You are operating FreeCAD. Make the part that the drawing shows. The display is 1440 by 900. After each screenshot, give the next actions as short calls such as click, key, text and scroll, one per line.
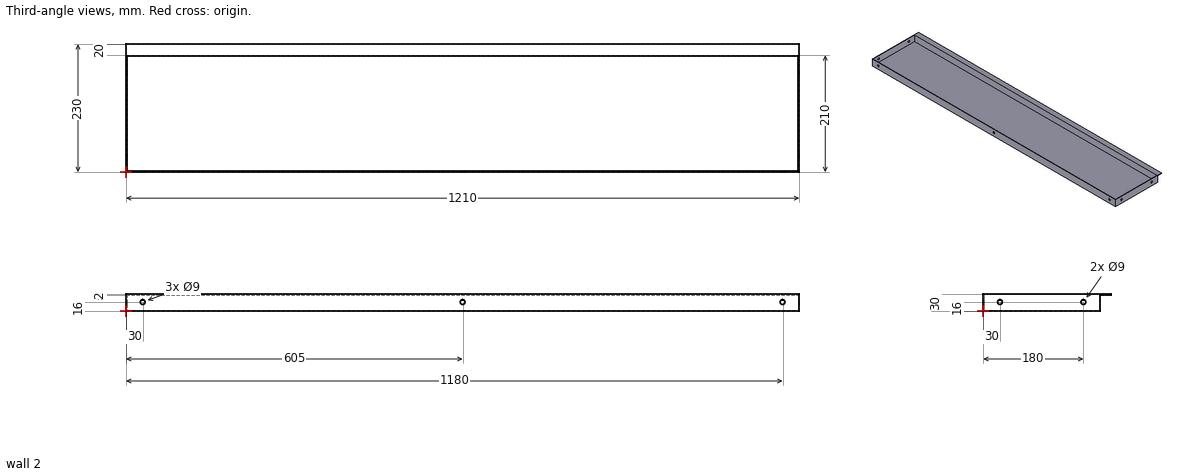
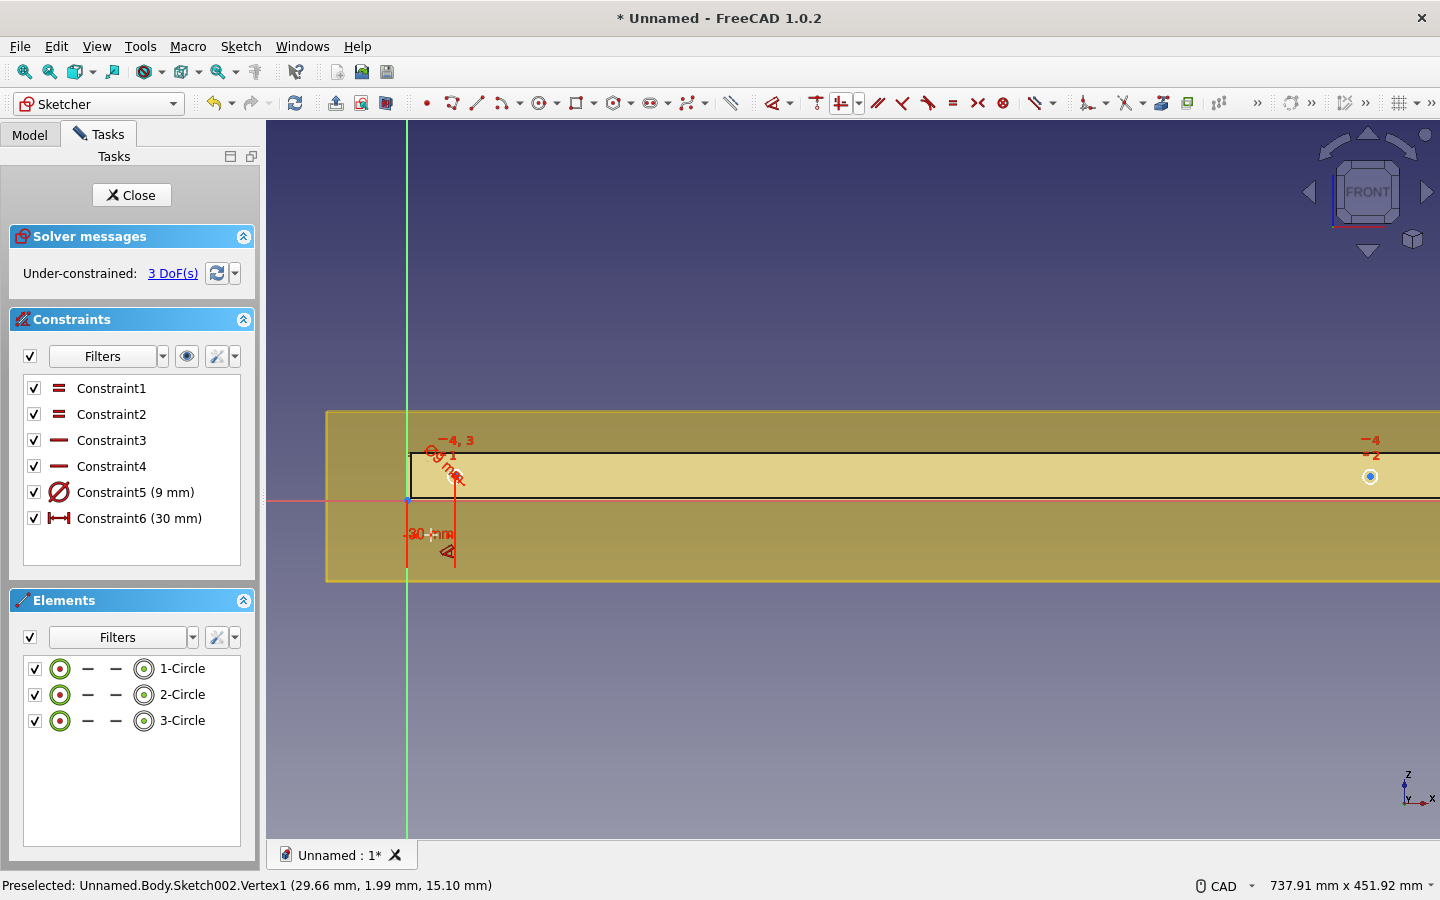
scroll(455, 477, up, 3)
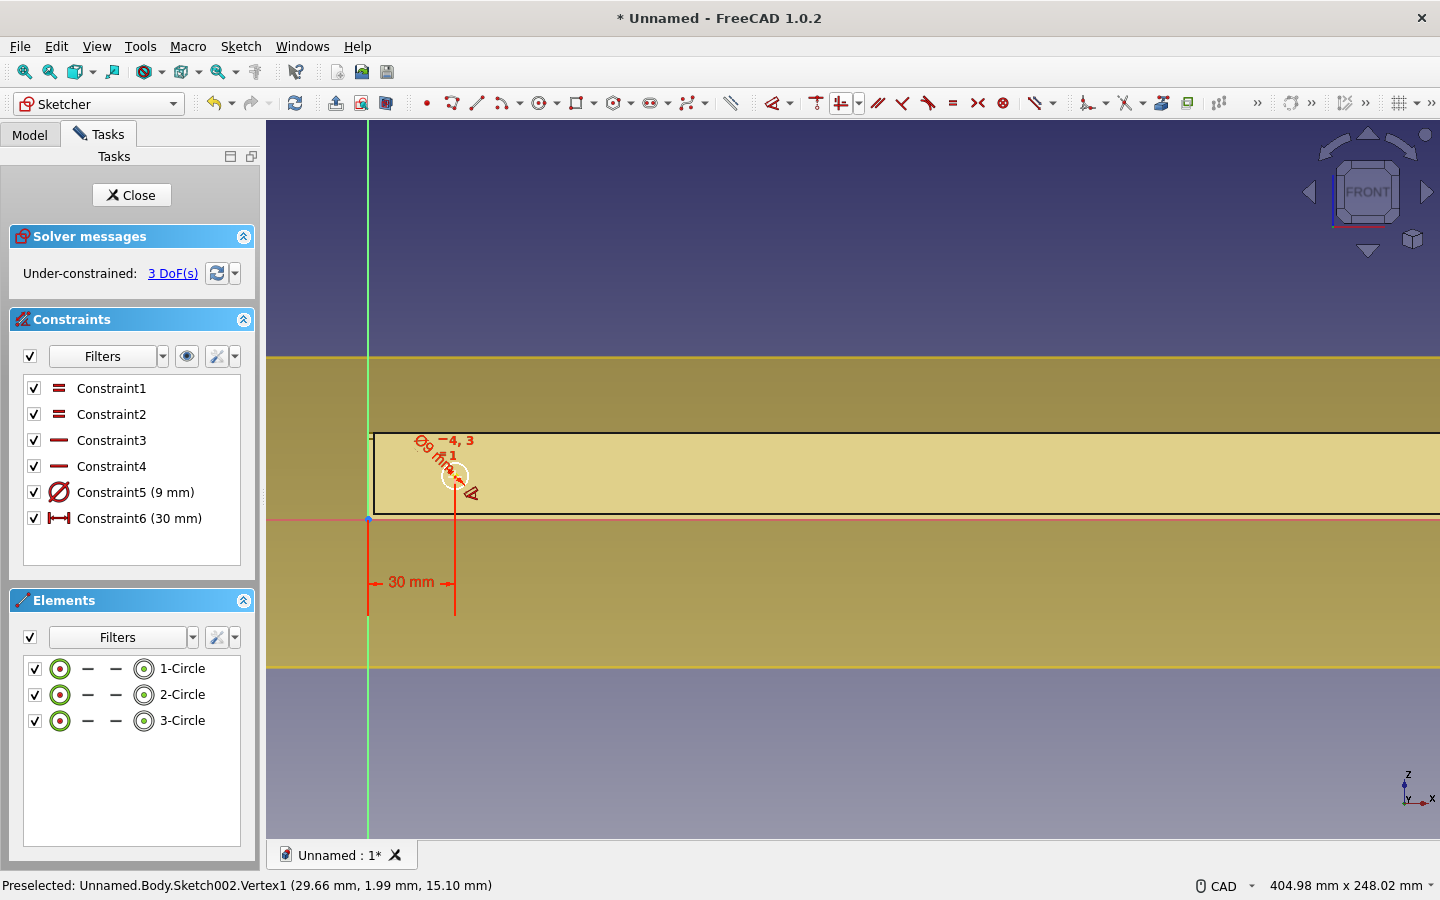
click(455, 476)
click(334, 498)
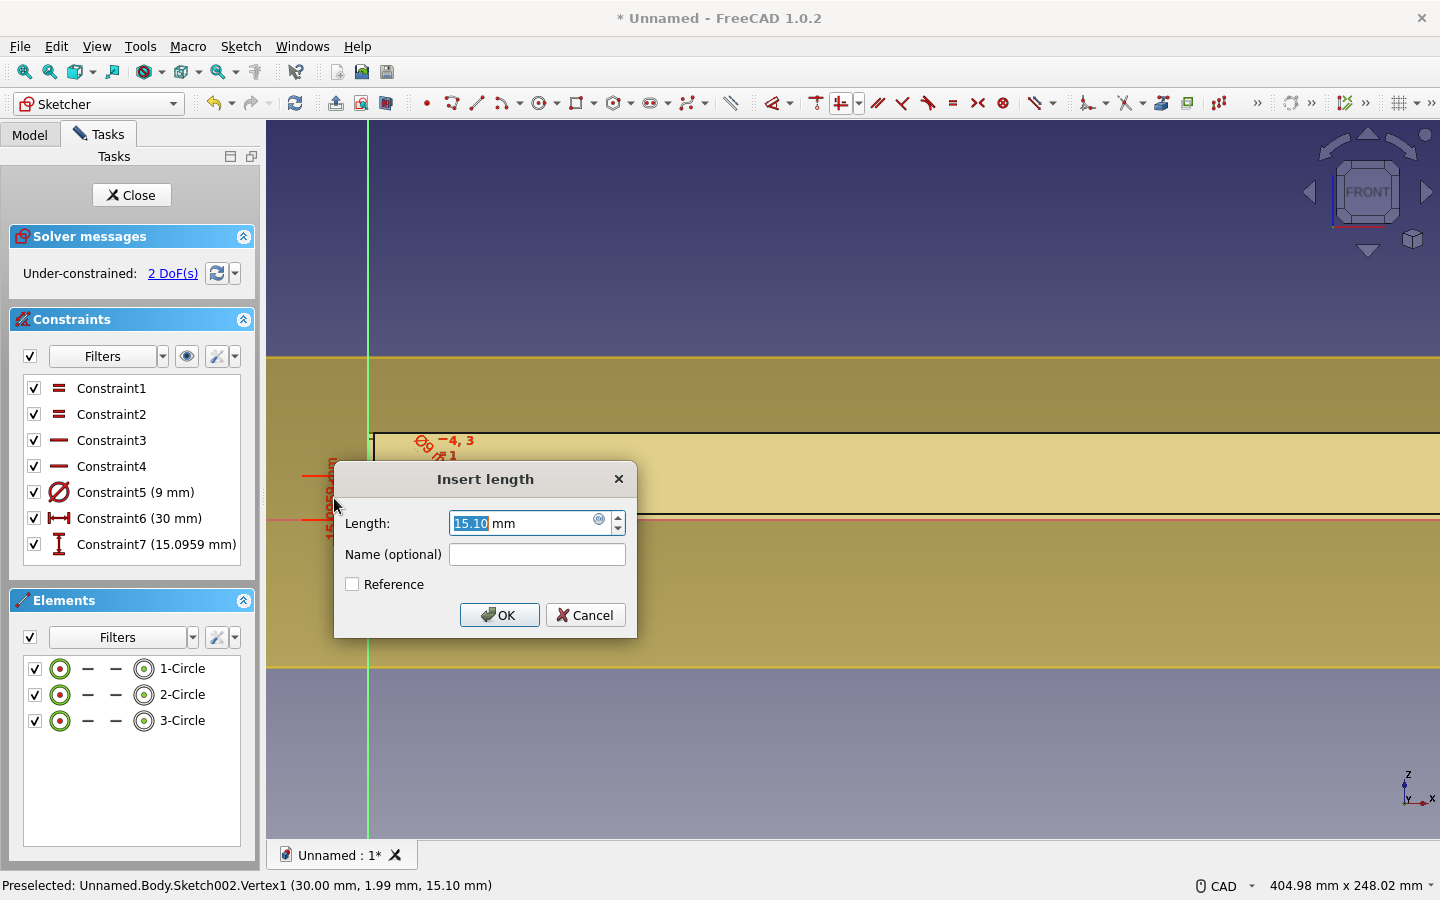
text(16)
key(Return)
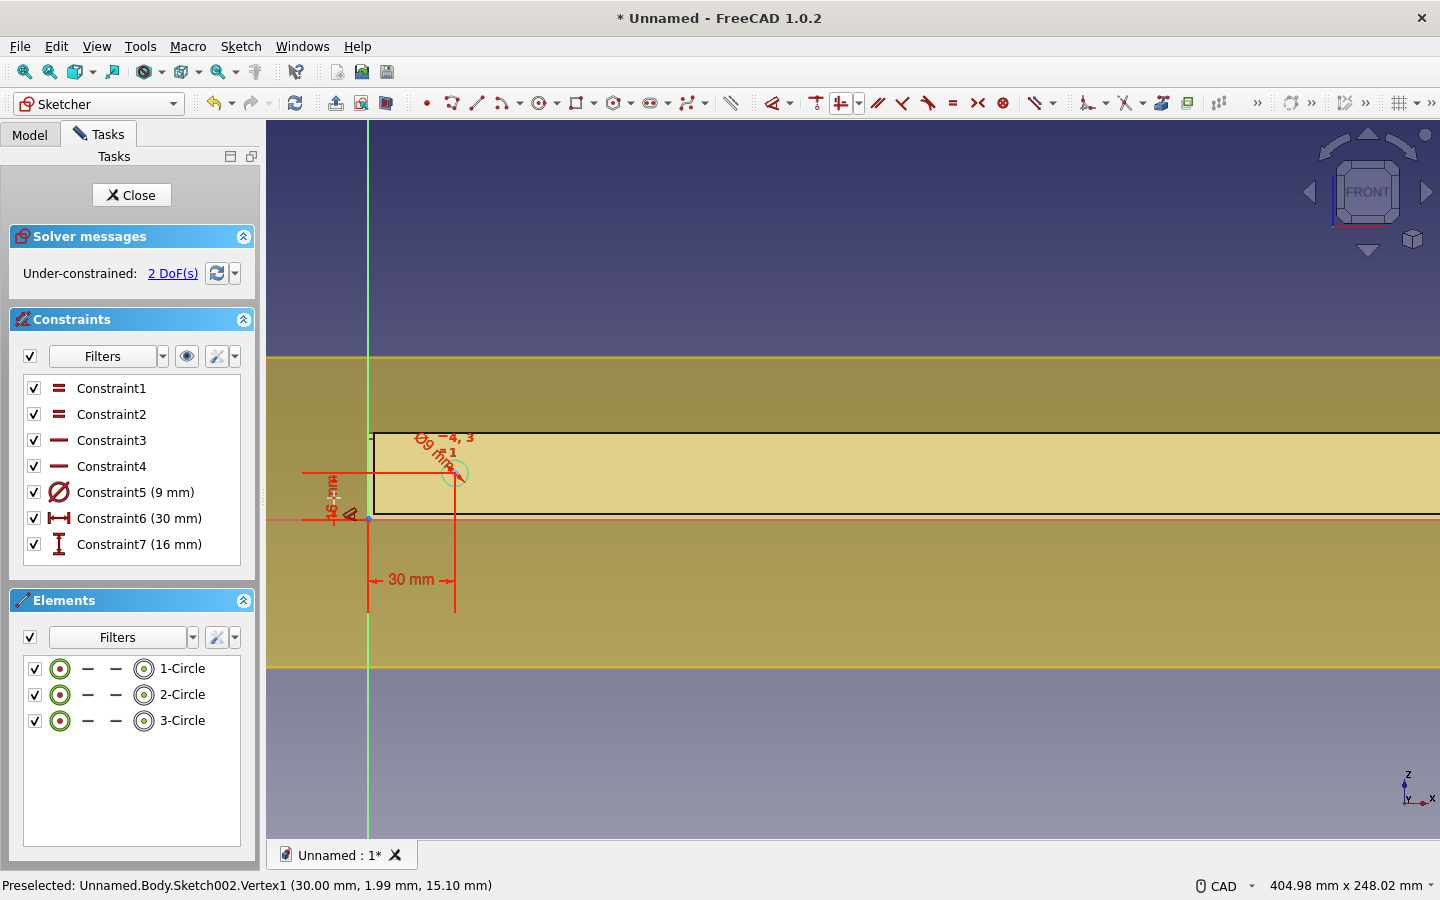
scroll(455, 477, down, 8)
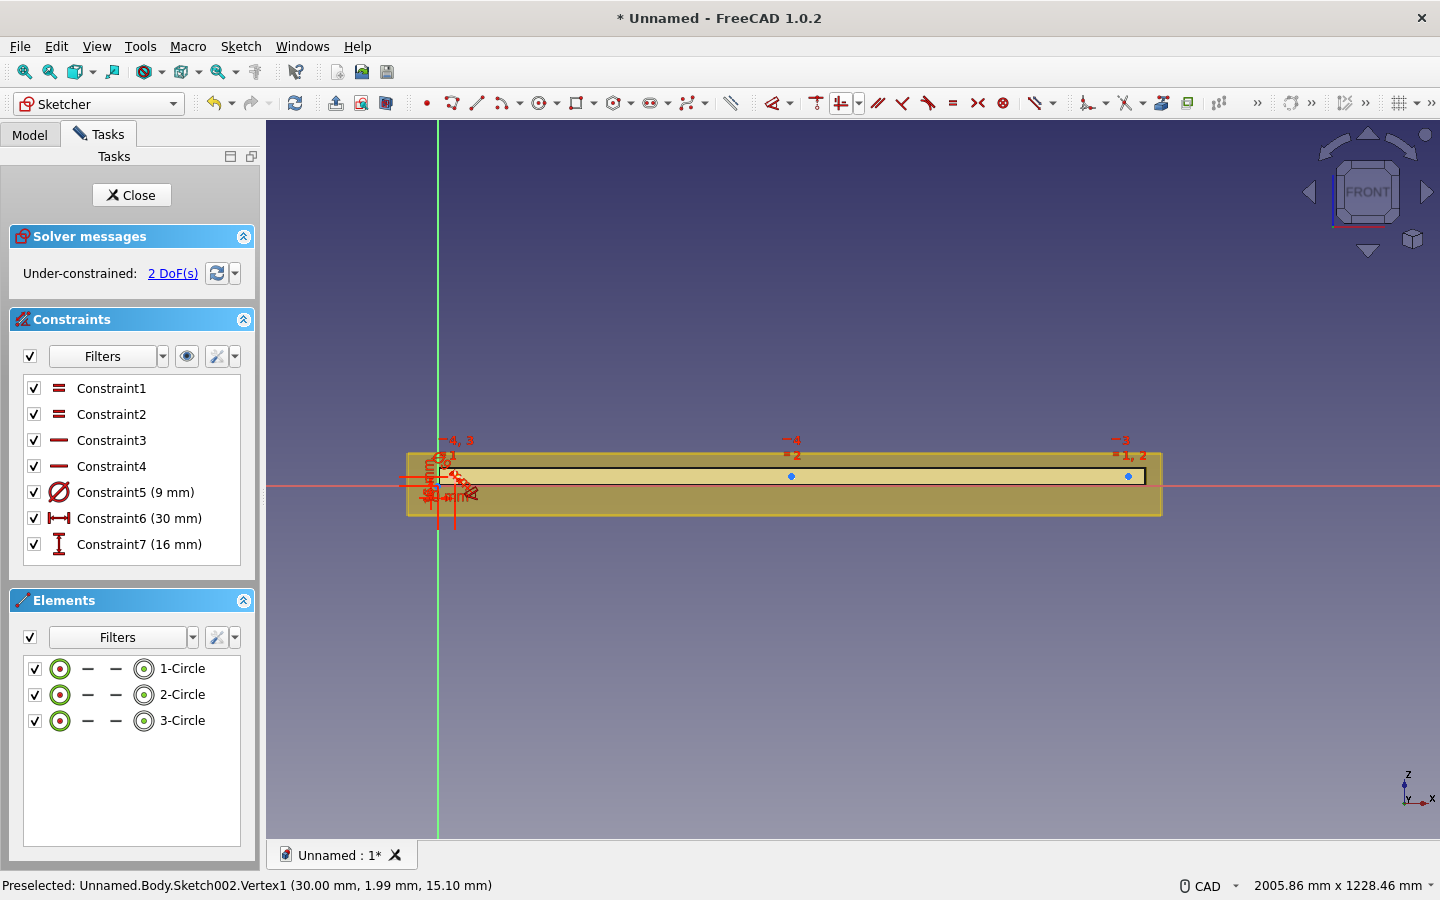
click(792, 477)
click(615, 520)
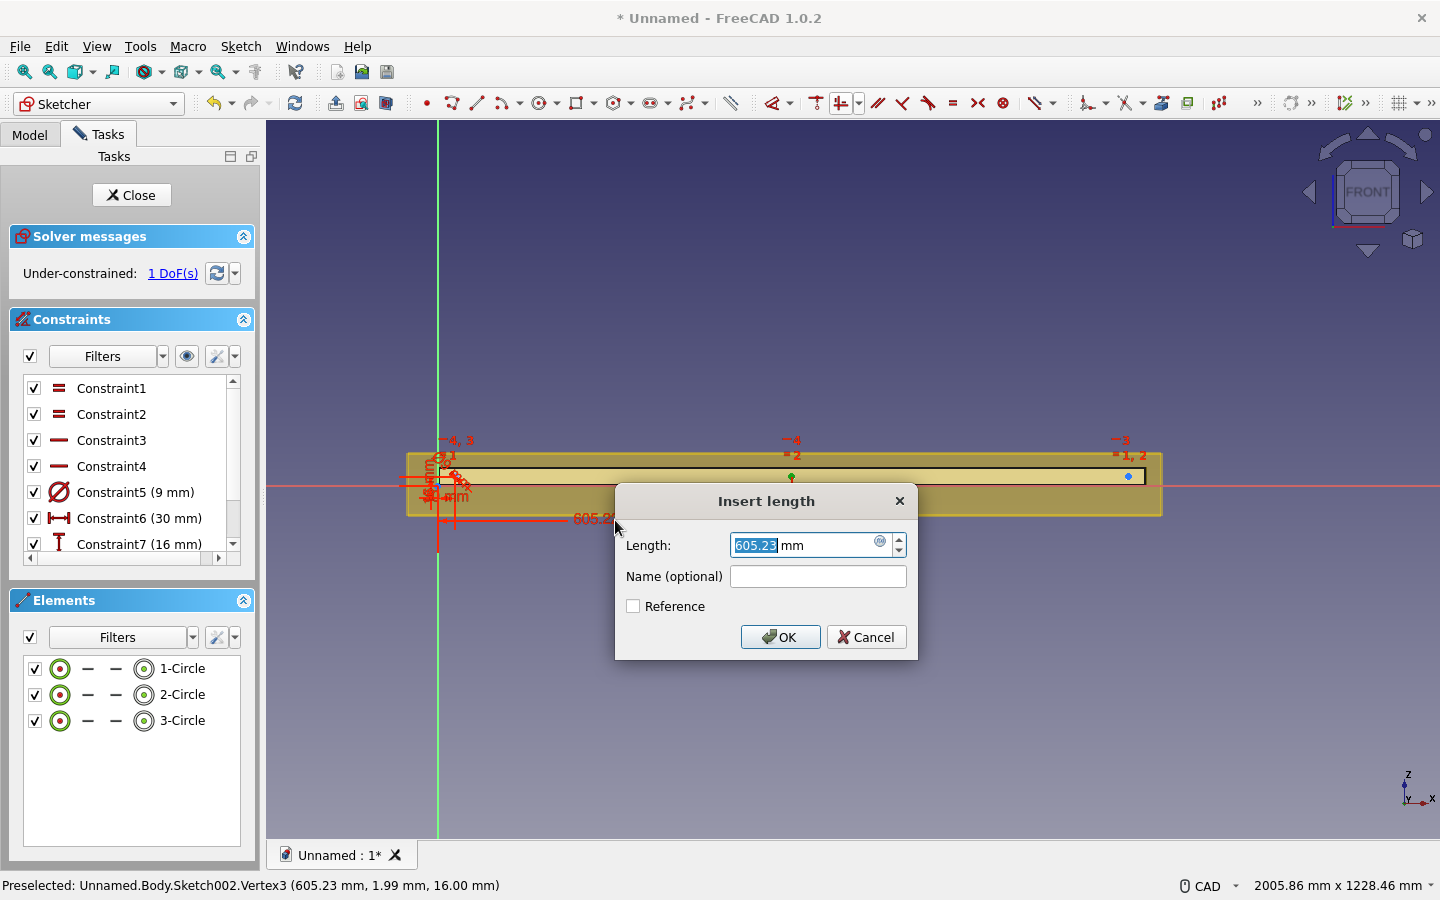
text(605)
key(Return)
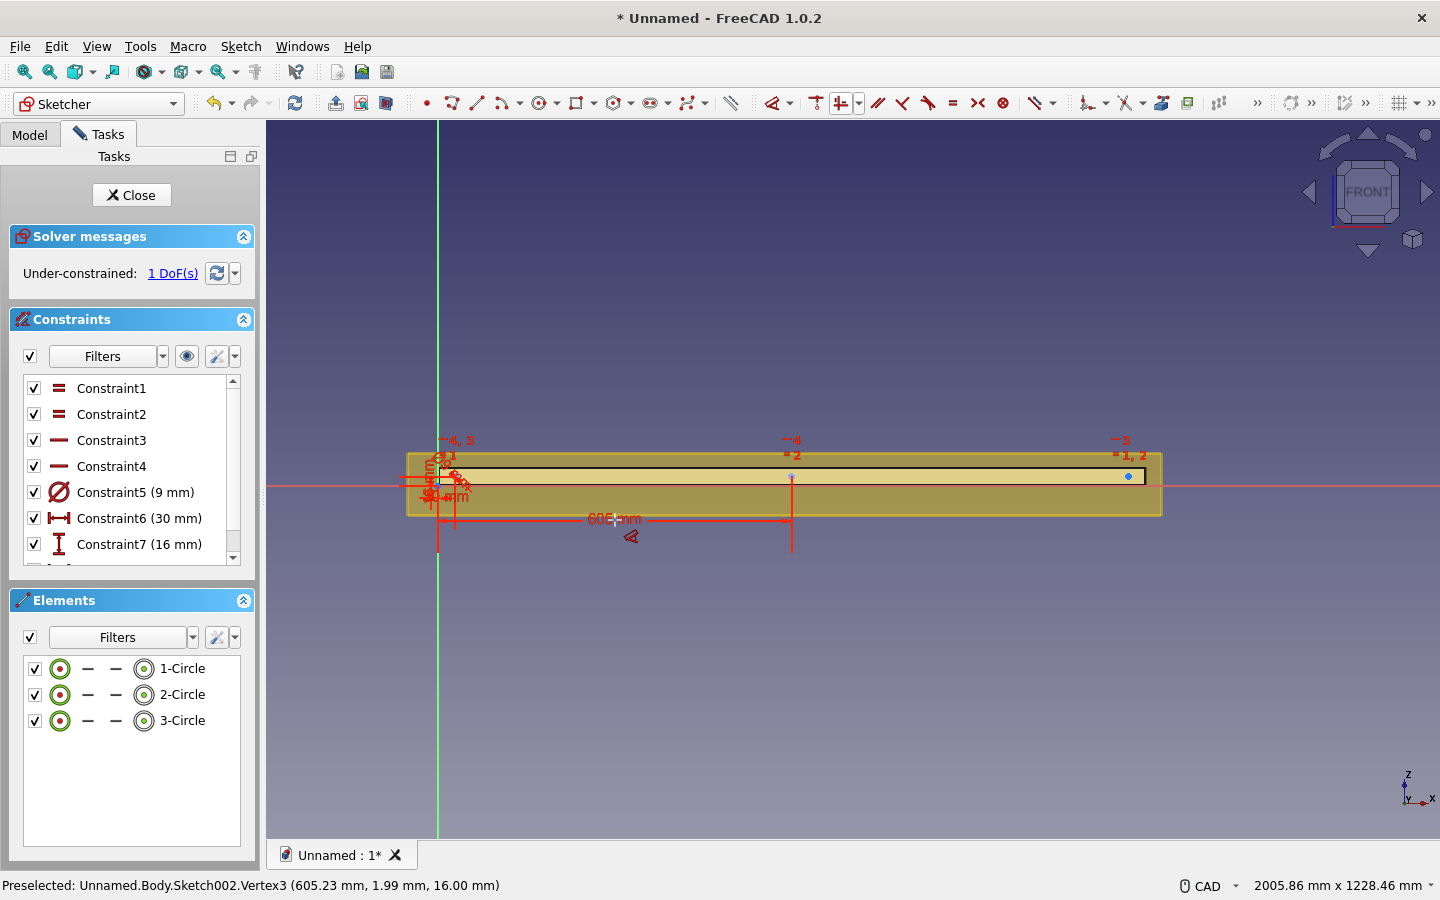
click(1128, 477)
click(783, 520)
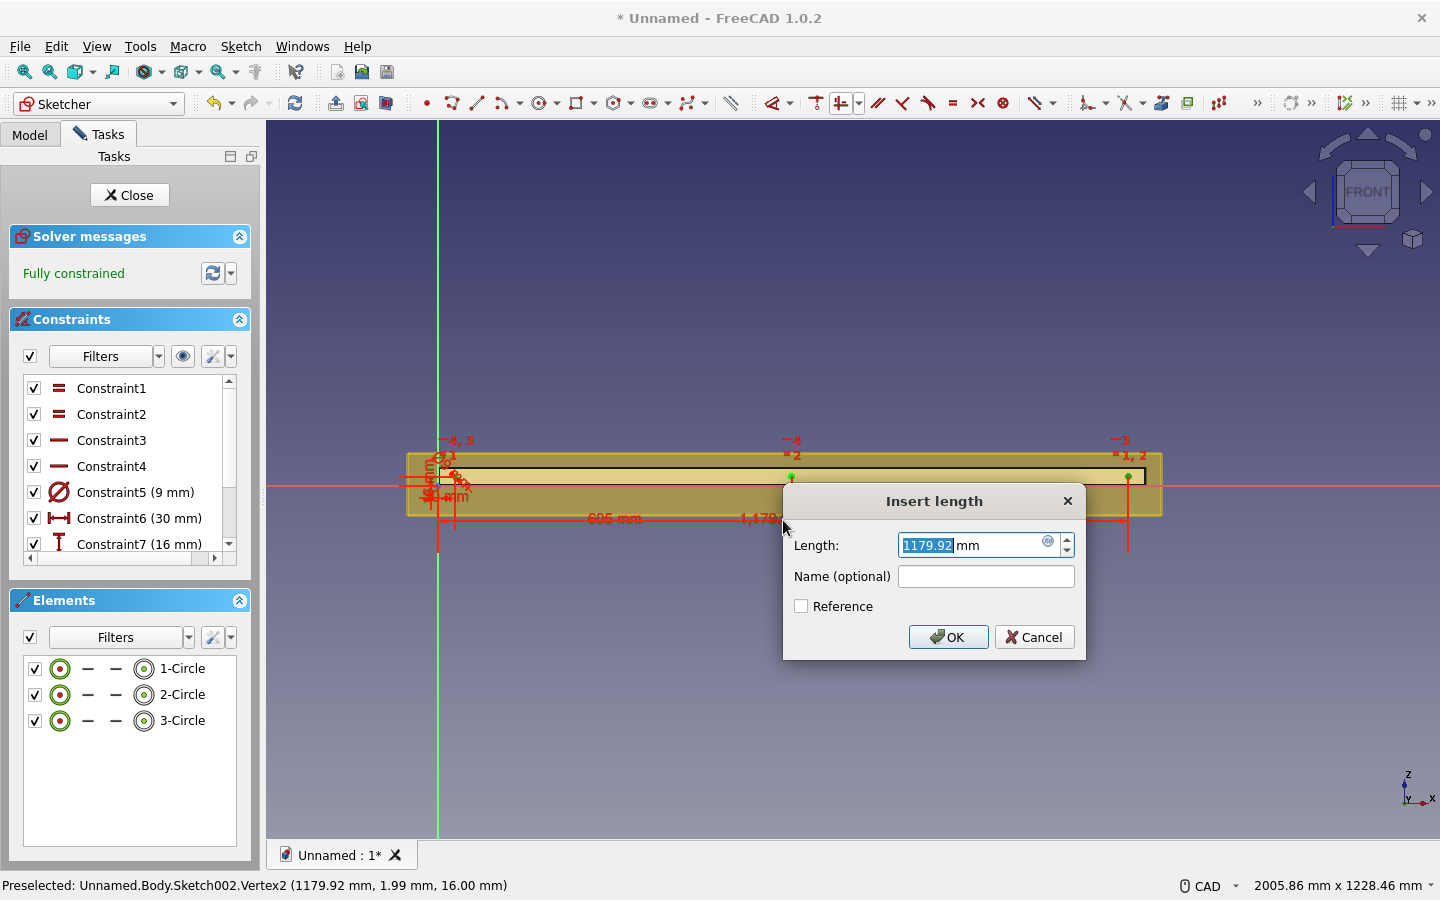
text(1180)
key(Return)
key(Escape)